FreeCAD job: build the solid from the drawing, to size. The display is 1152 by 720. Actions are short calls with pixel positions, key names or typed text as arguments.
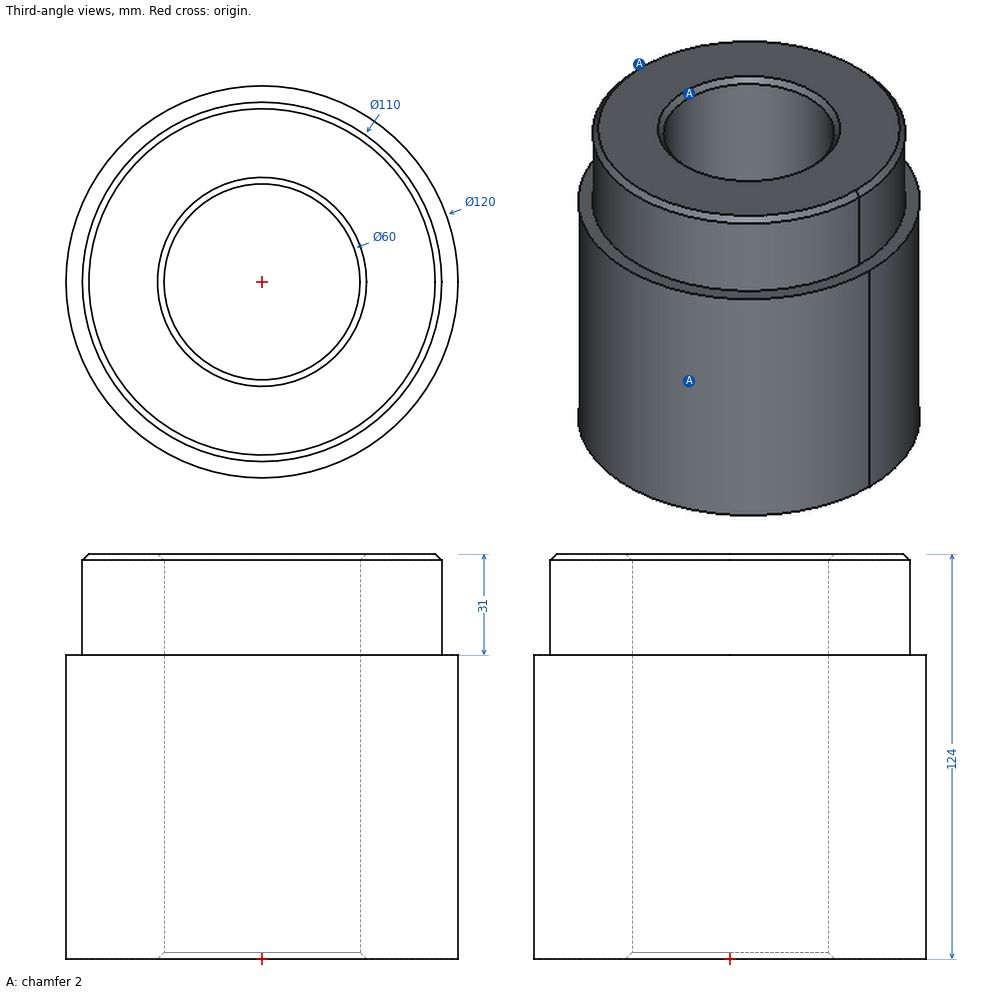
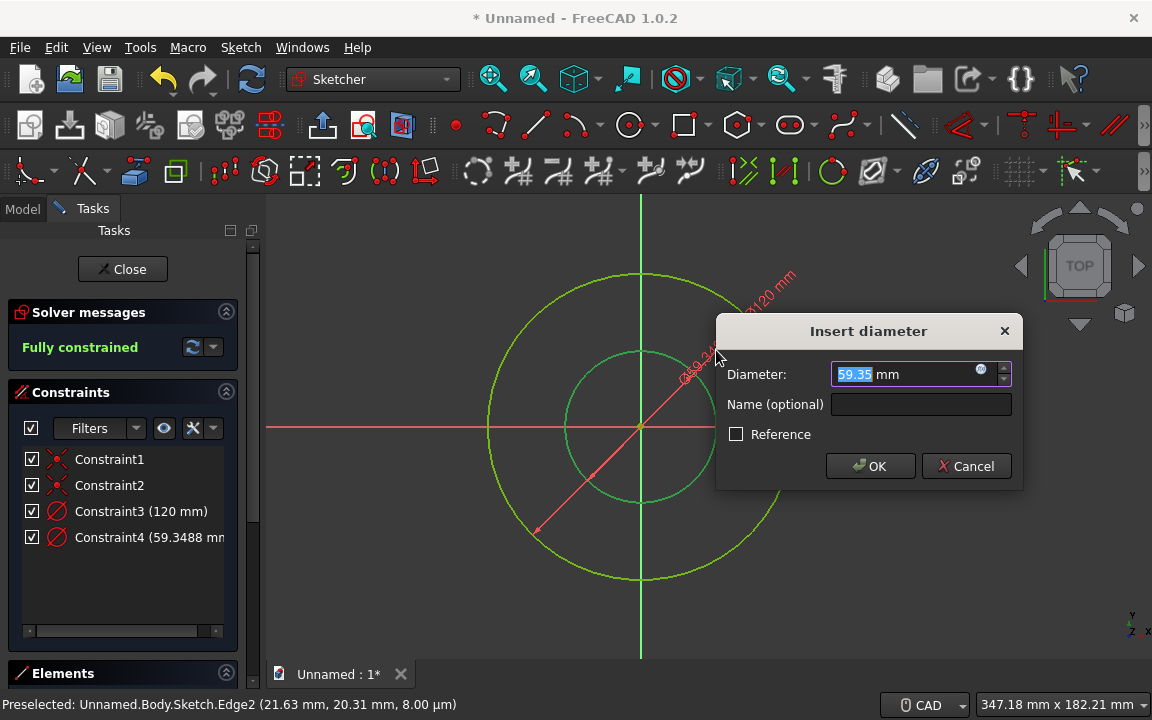
text(60)
key(Return)
key(Escape)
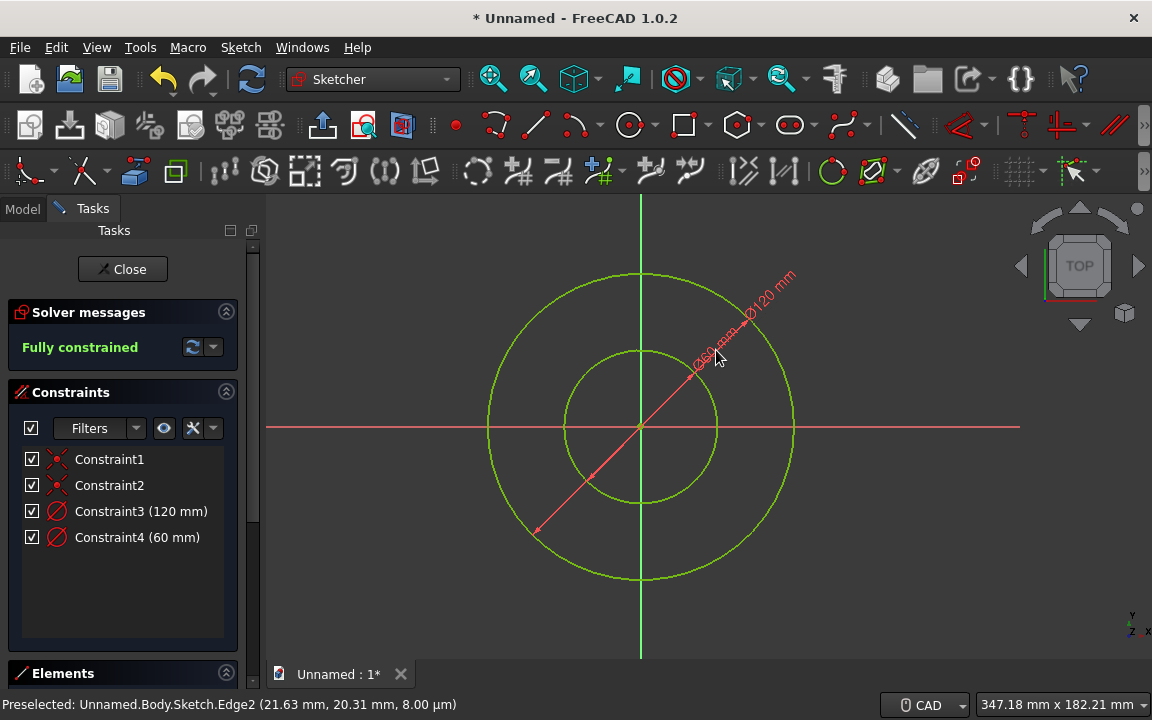
click(123, 269)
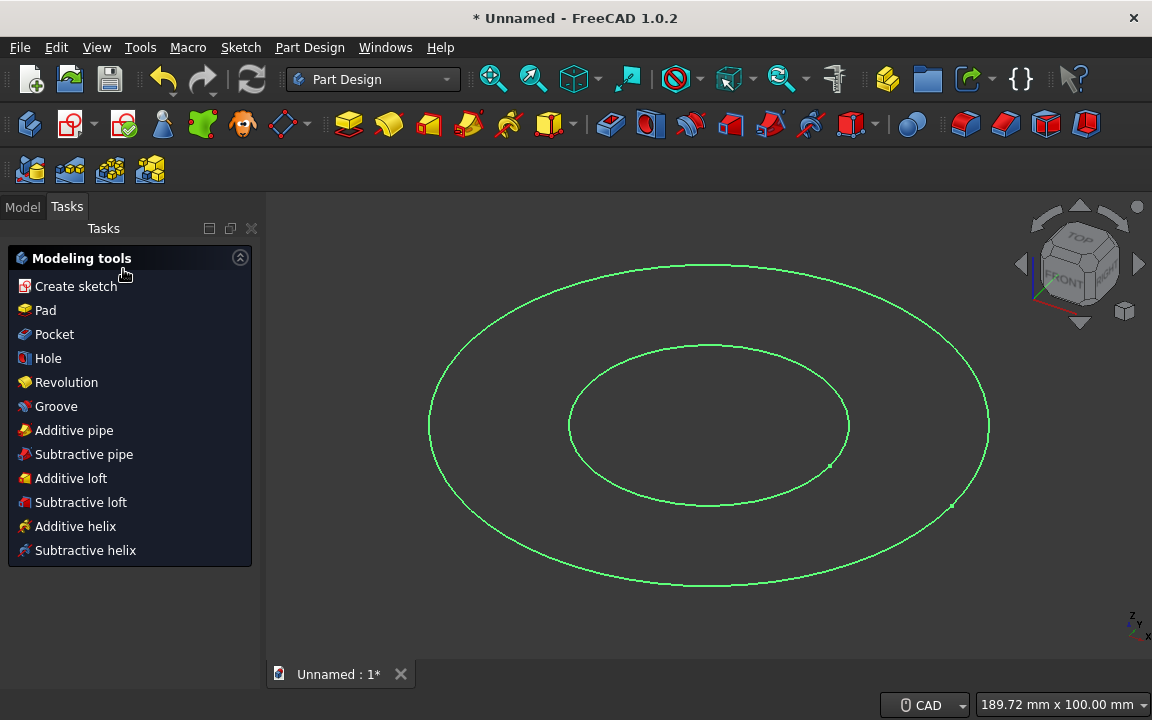
click(350, 124)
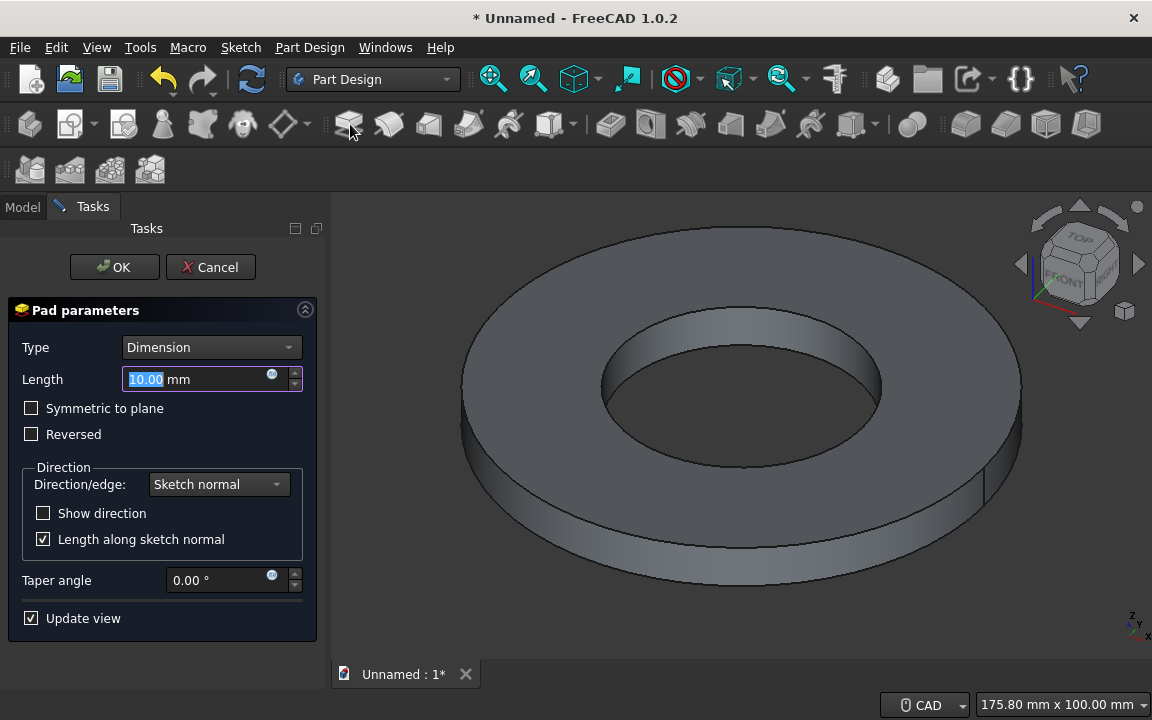
text(124)
key(Tab)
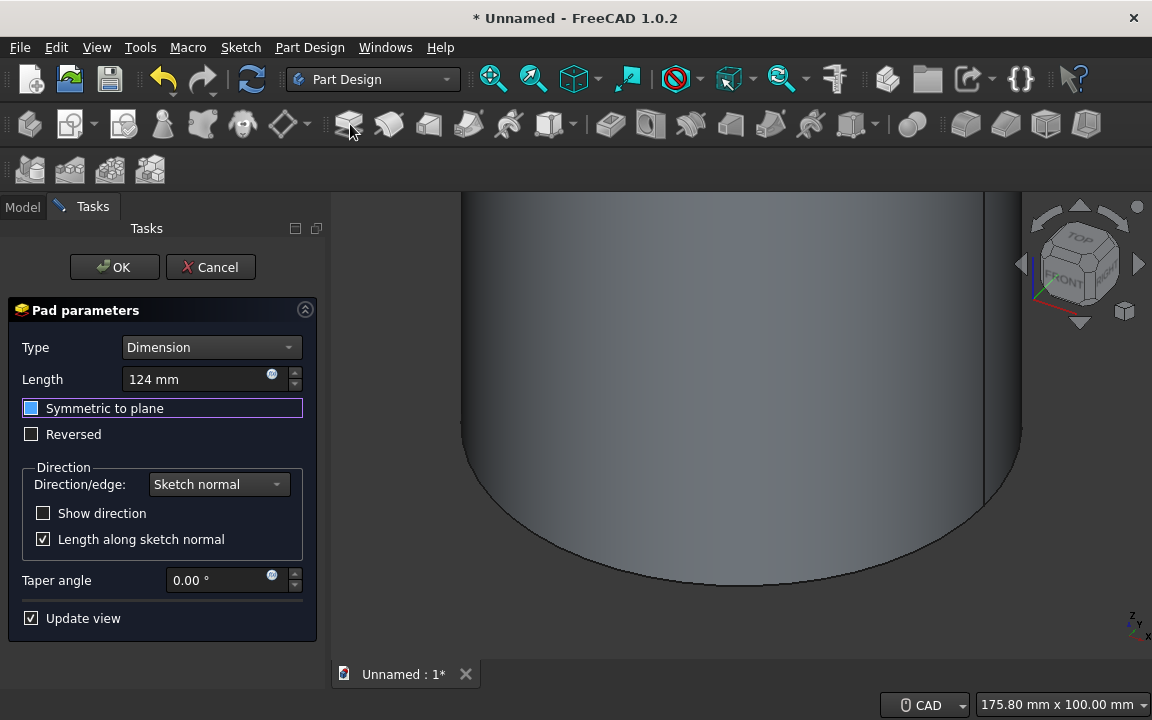
click(115, 267)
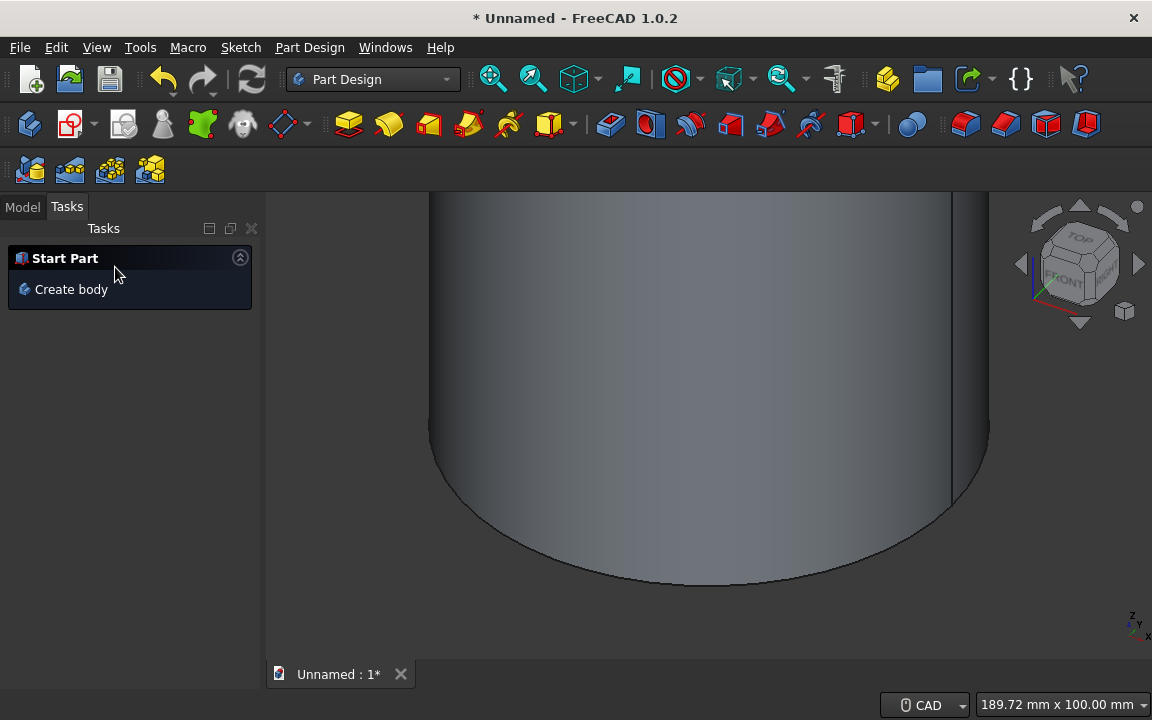
click(494, 80)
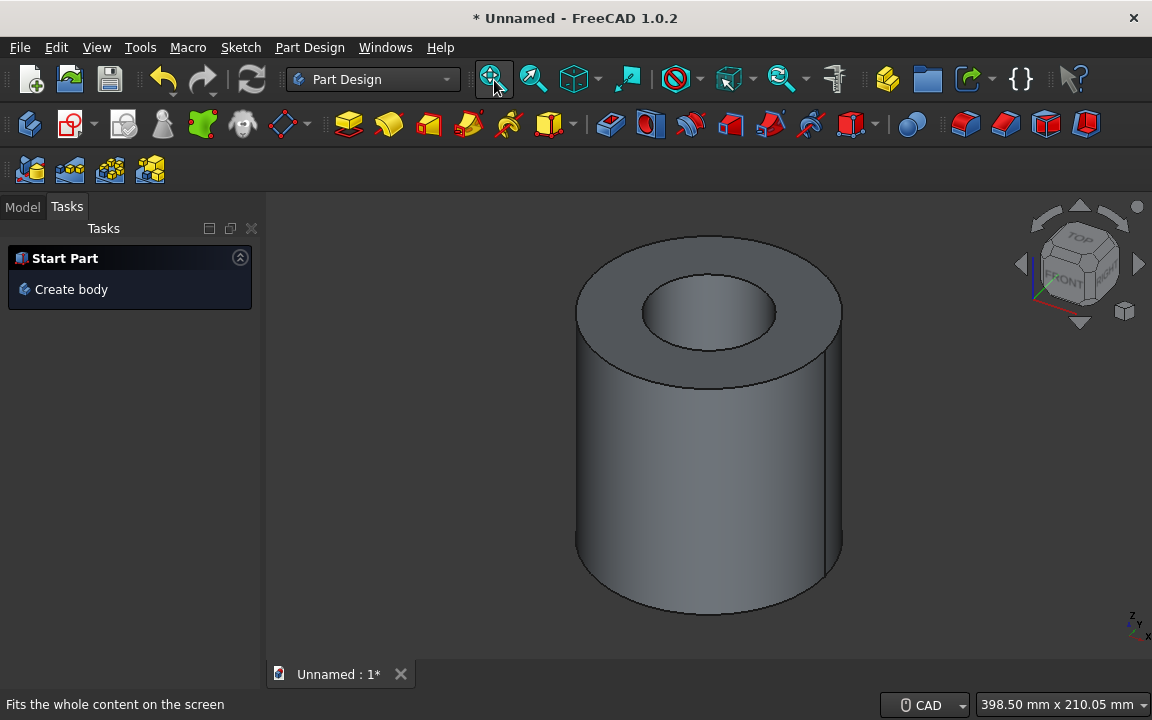
click(23, 206)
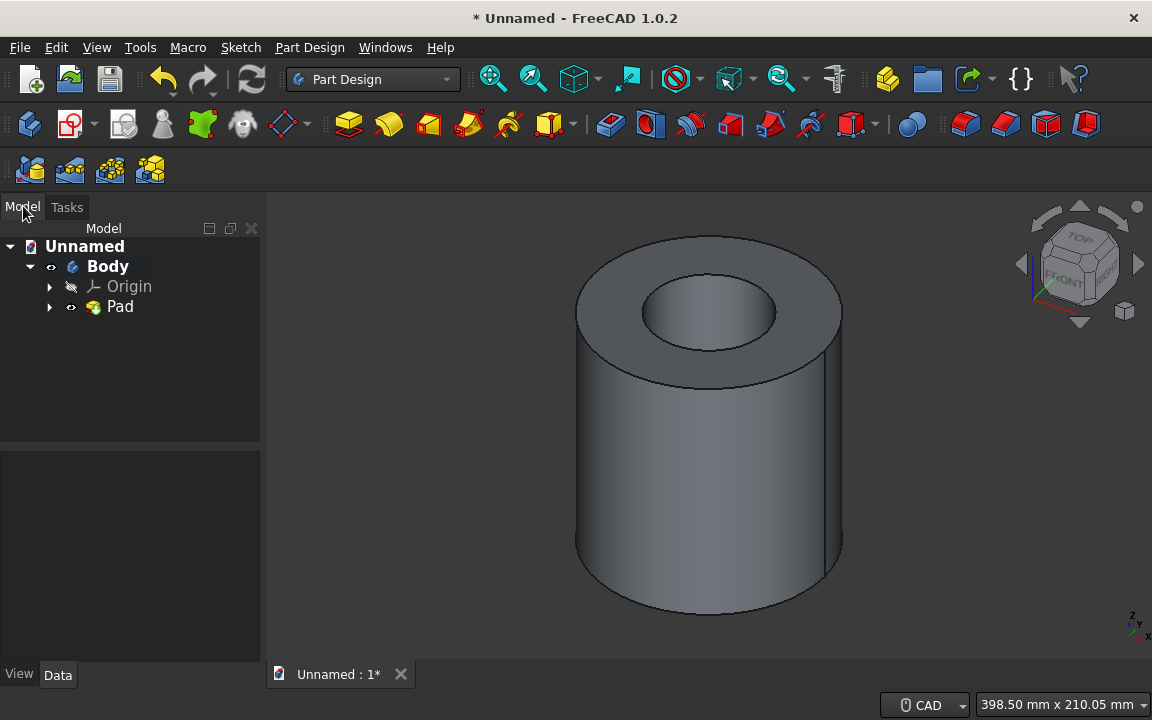
click(50, 287)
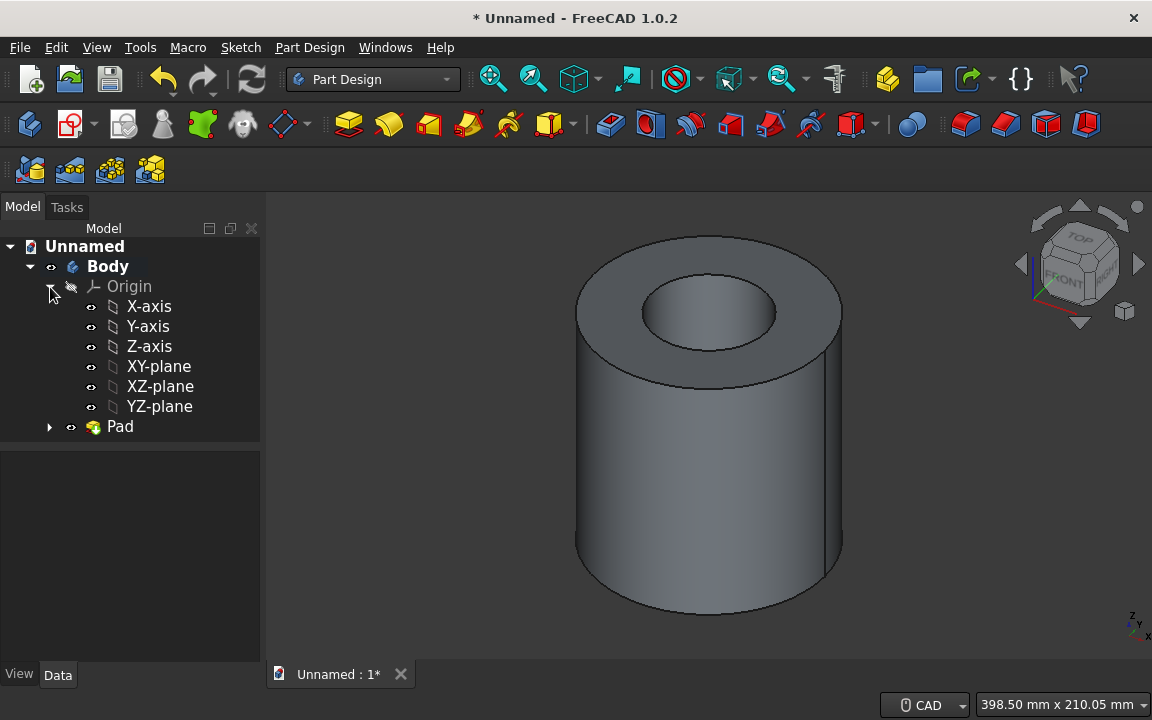
click(136, 367)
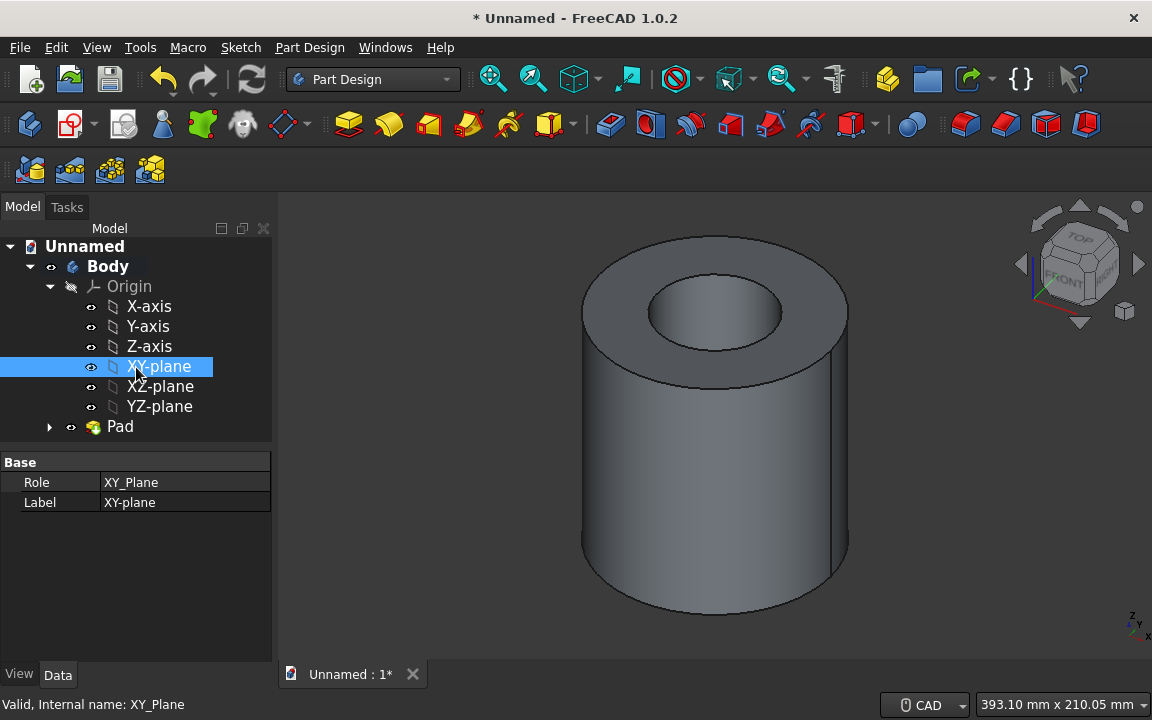
click(284, 124)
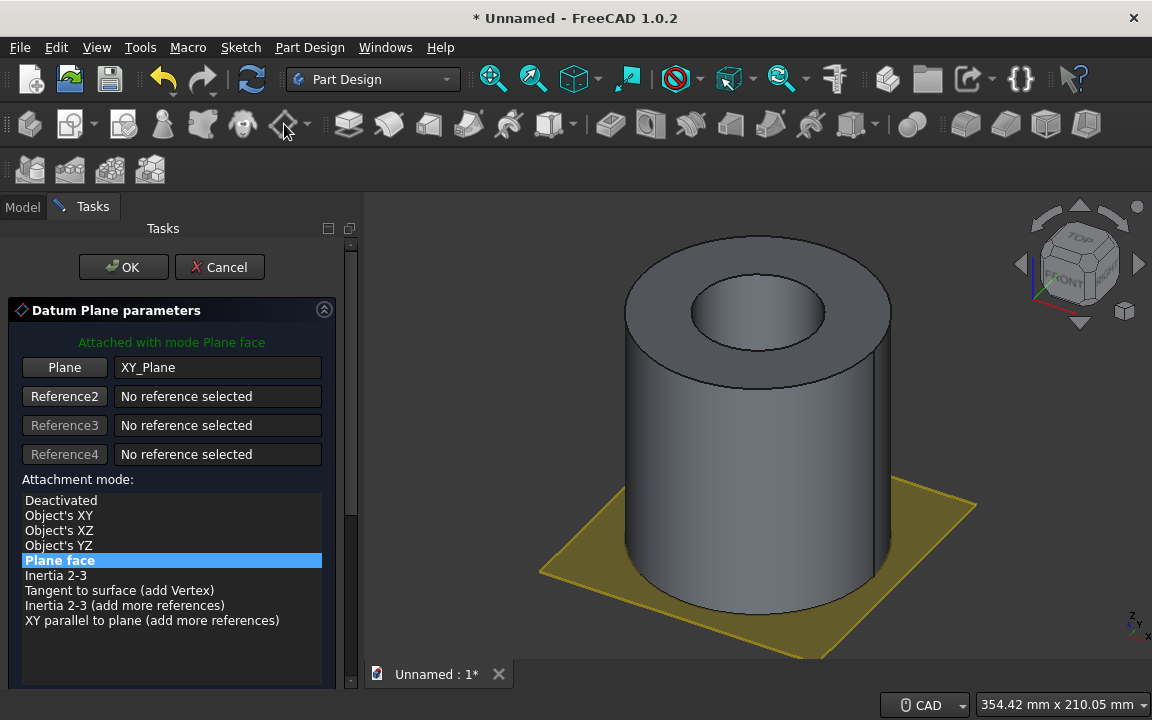
scroll(351, 463, down, 3)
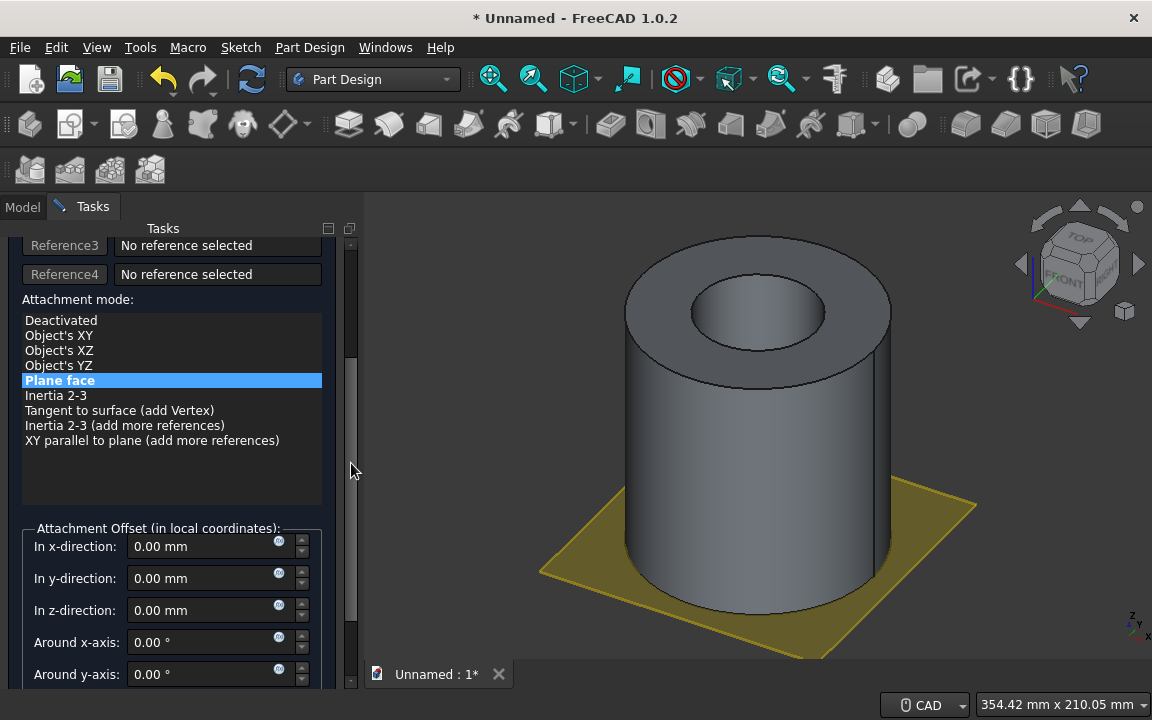
triple_click(210, 610)